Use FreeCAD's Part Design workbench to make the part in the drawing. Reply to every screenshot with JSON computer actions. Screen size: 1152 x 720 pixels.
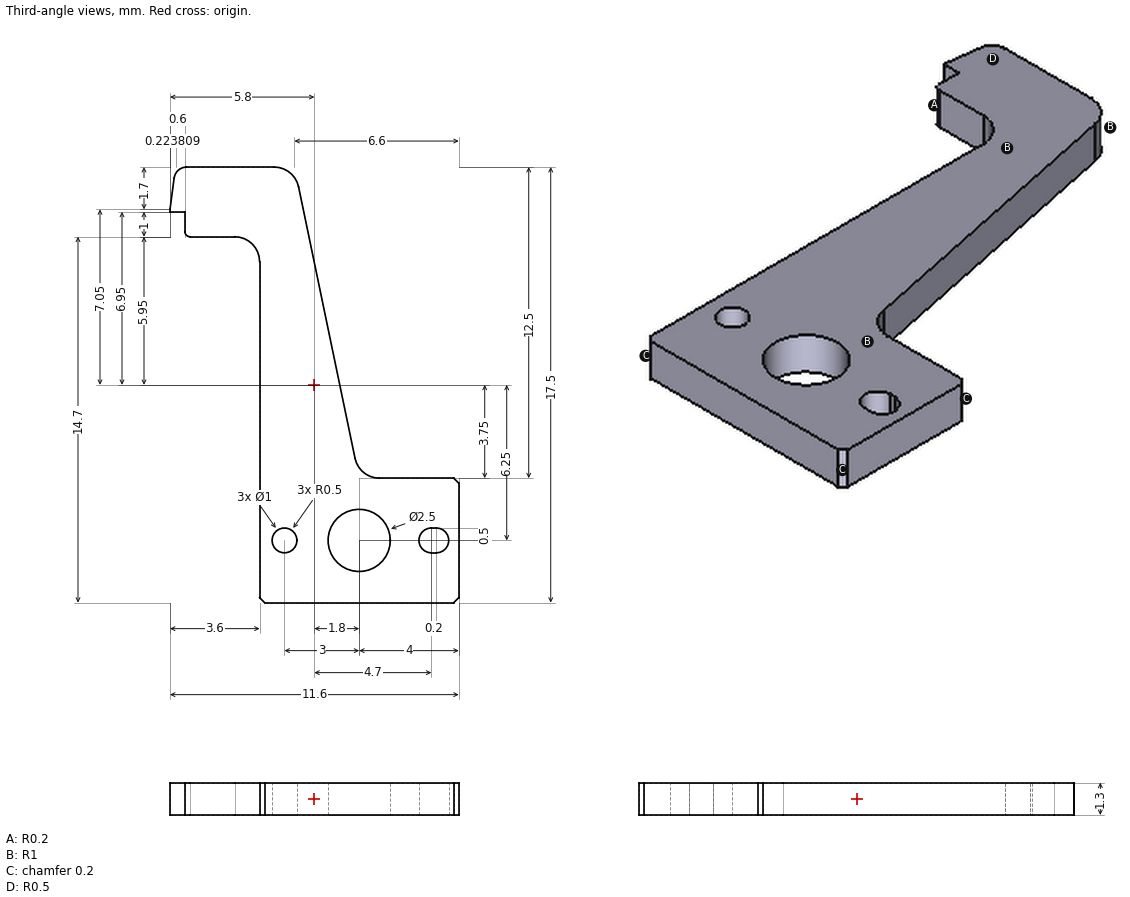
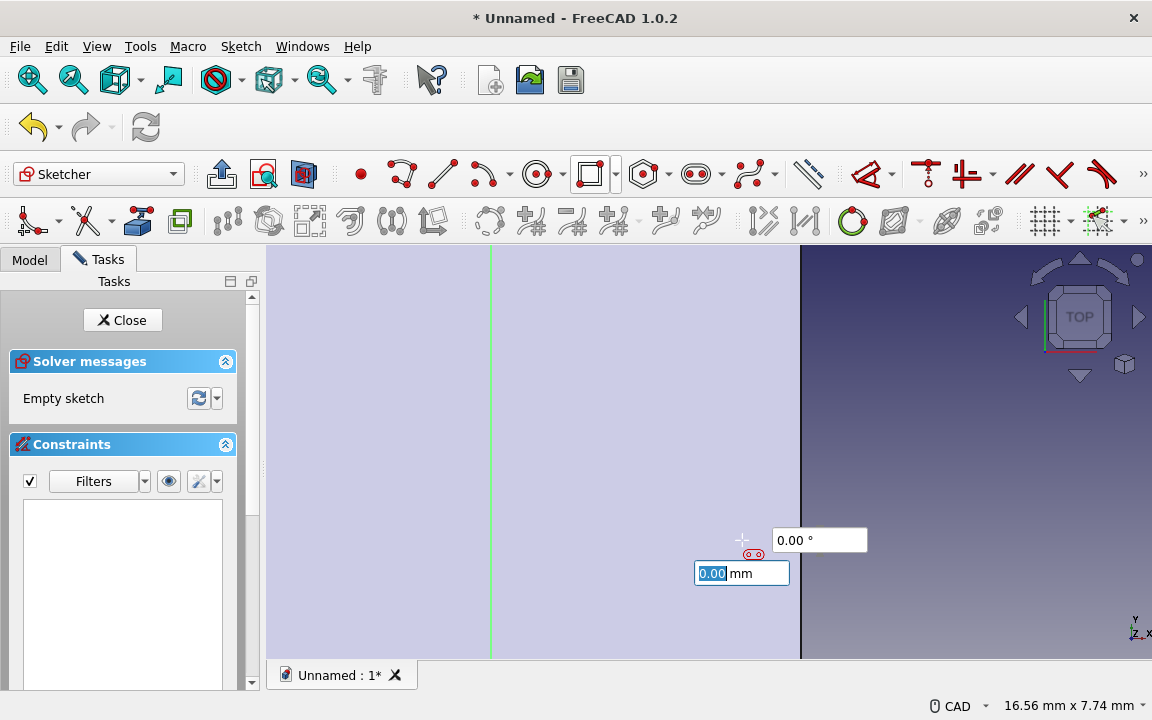
{"action": "scroll", "coordinate": [753, 540], "scroll_direction": "up", "scroll_amount": 2}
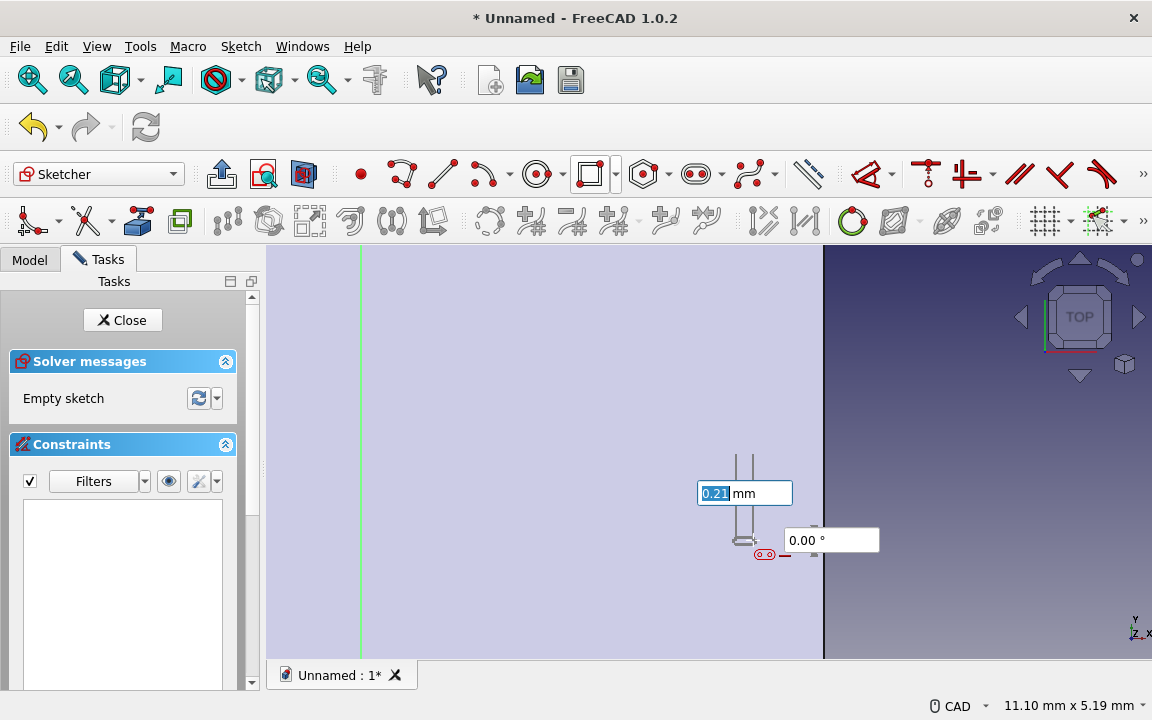
{"action": "left_click", "coordinate": [752, 540]}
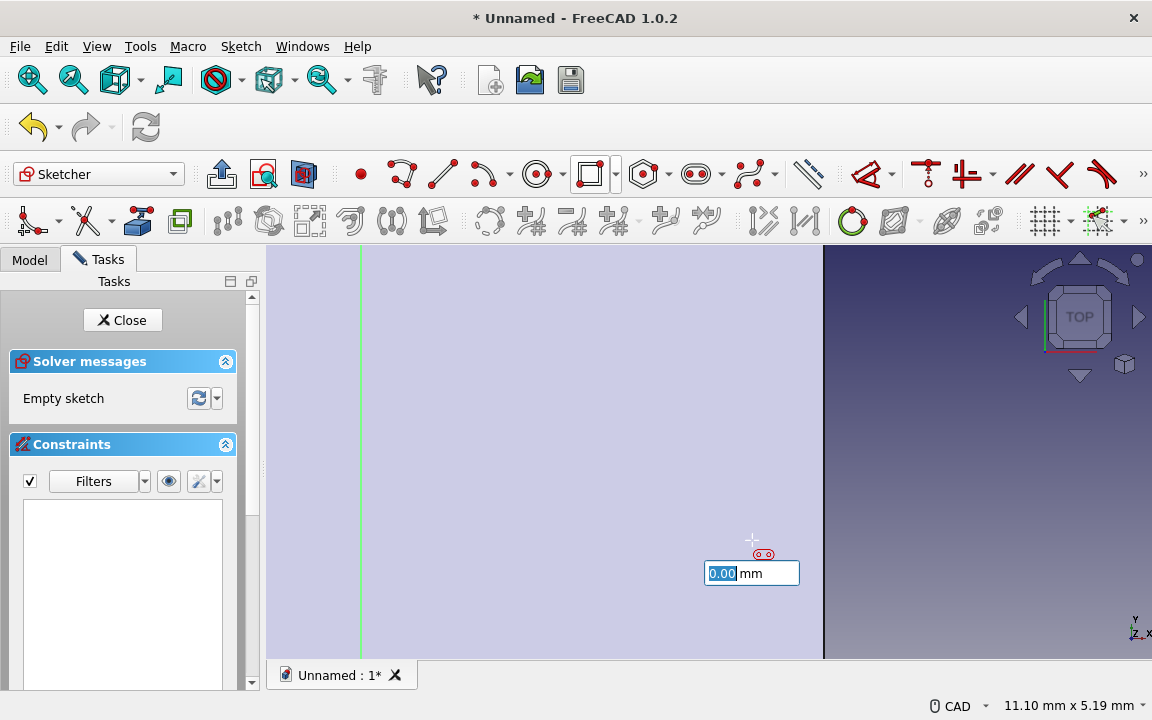
{"action": "left_click", "coordinate": [744, 500]}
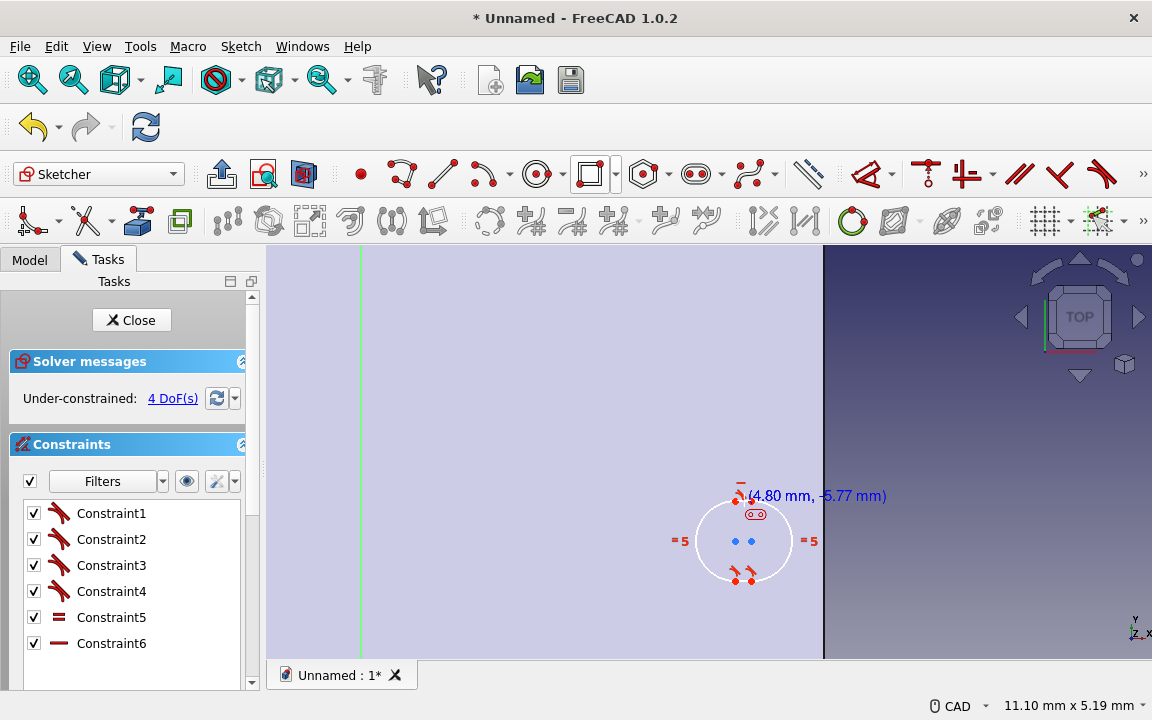
{"action": "left_click", "coordinate": [536, 174]}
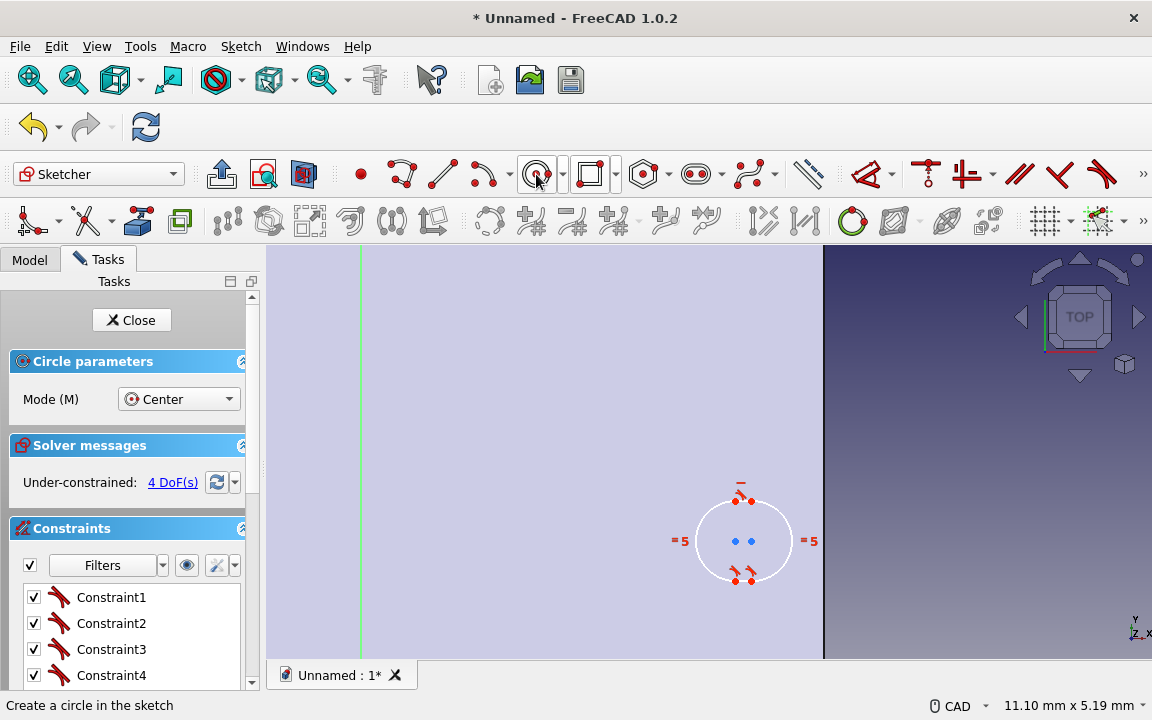
{"action": "left_click", "coordinate": [505, 540]}
{"action": "left_click", "coordinate": [575, 469]}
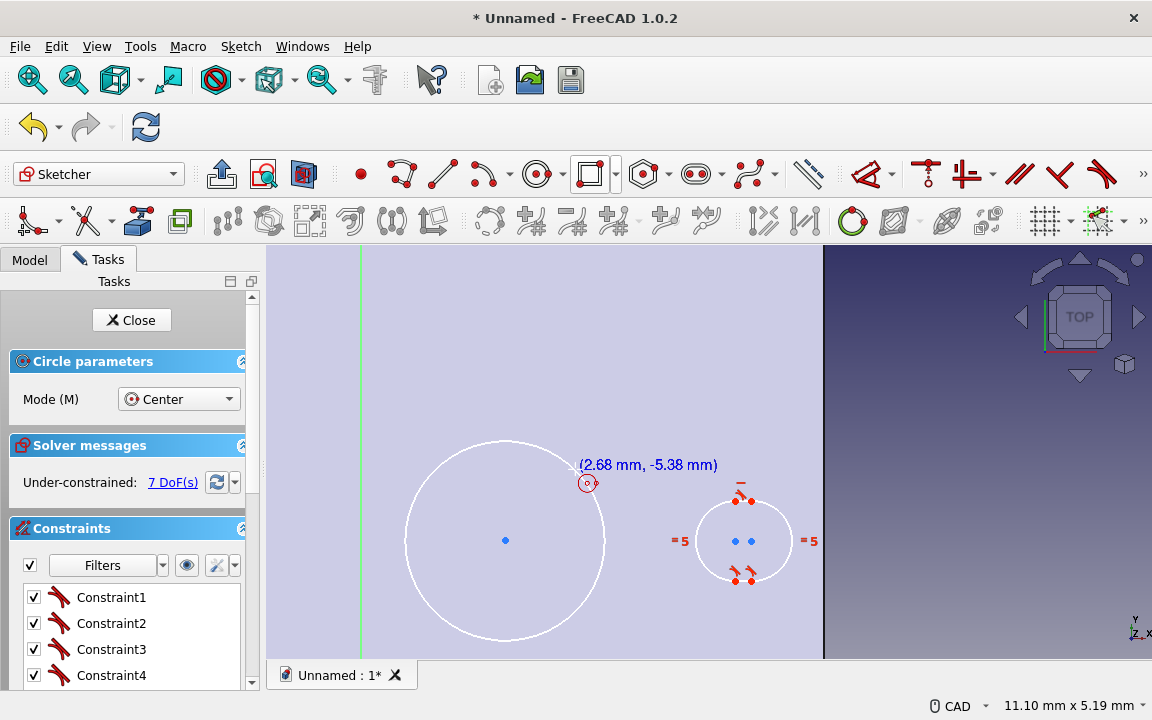
{"action": "scroll", "coordinate": [748, 543], "scroll_direction": "down", "scroll_amount": 4}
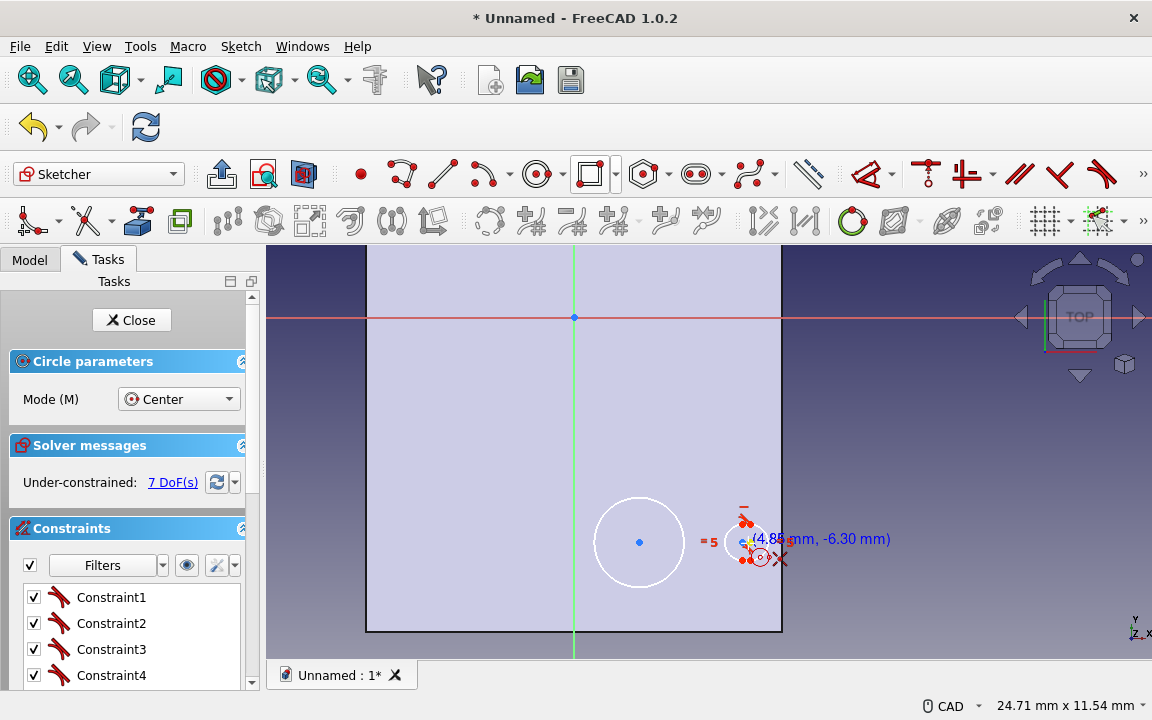
{"action": "scroll", "coordinate": [531, 542], "scroll_direction": "up", "scroll_amount": 2}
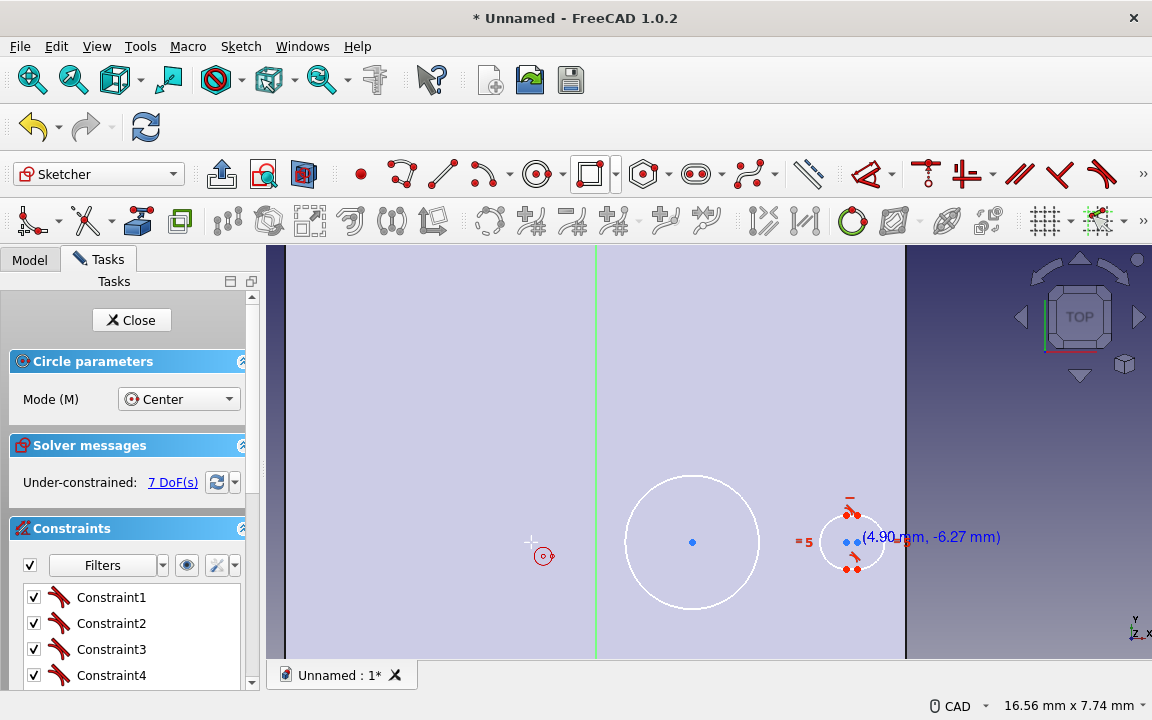
{"action": "left_click", "coordinate": [532, 541]}
{"action": "left_click", "coordinate": [550, 523]}
{"action": "key", "text": "Escape"}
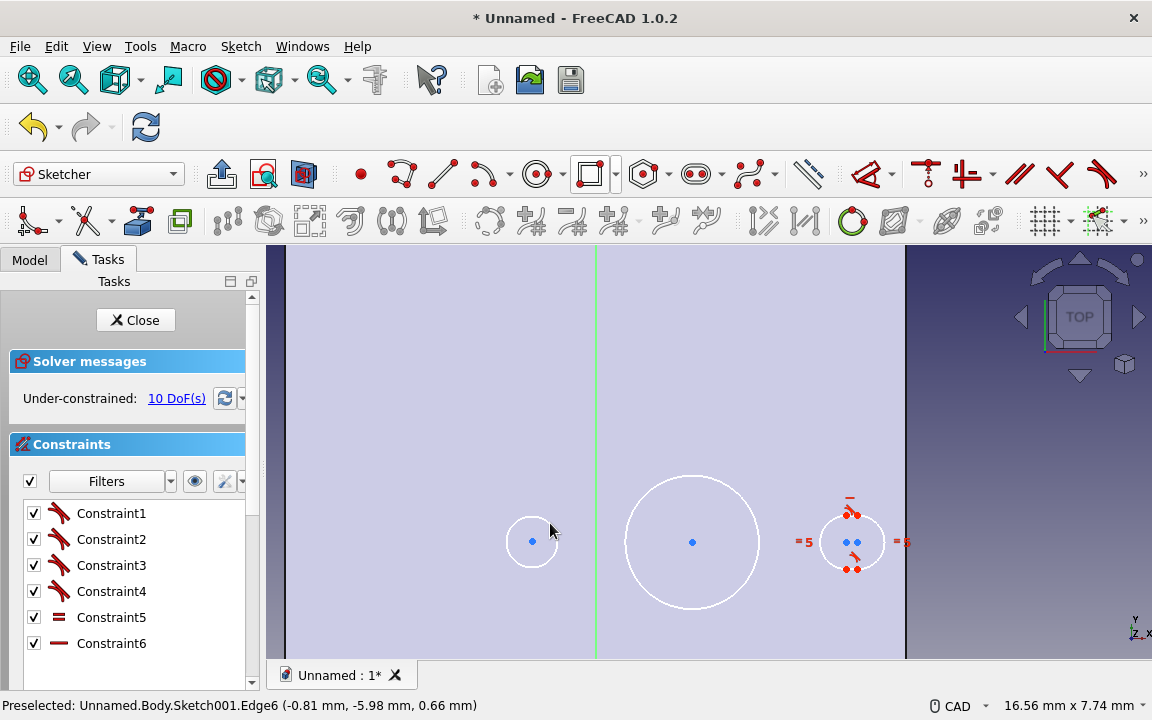
{"action": "left_click", "coordinate": [692, 542]}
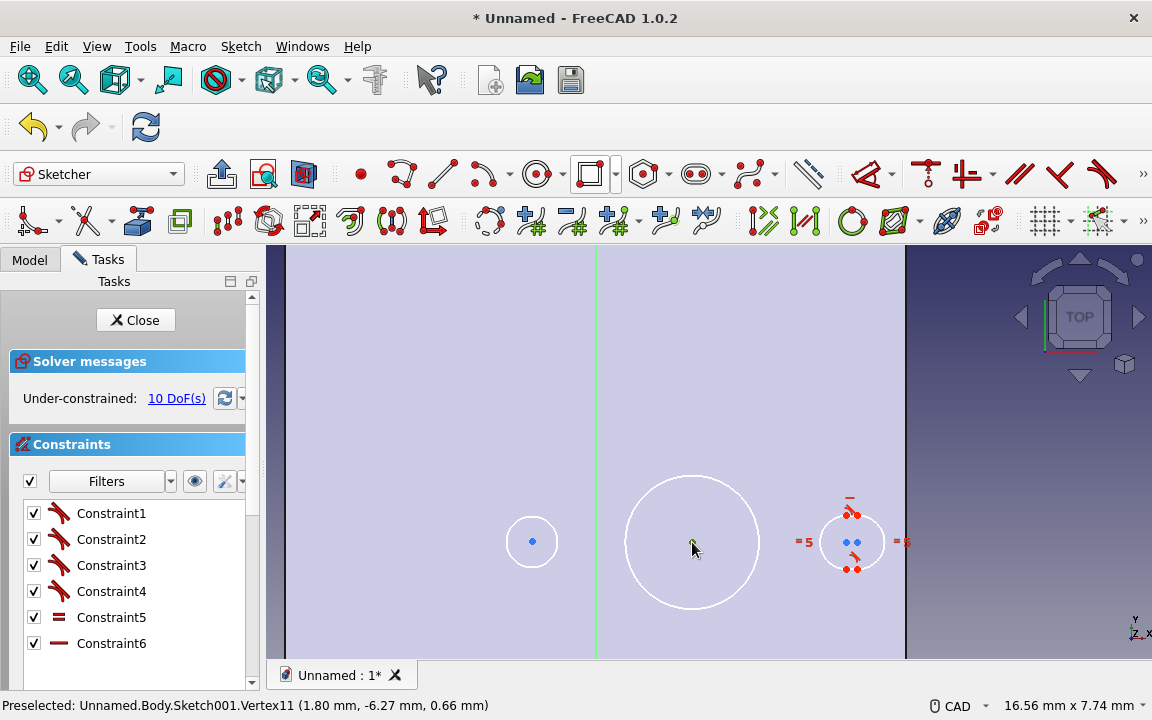
{"action": "left_click", "coordinate": [532, 542]}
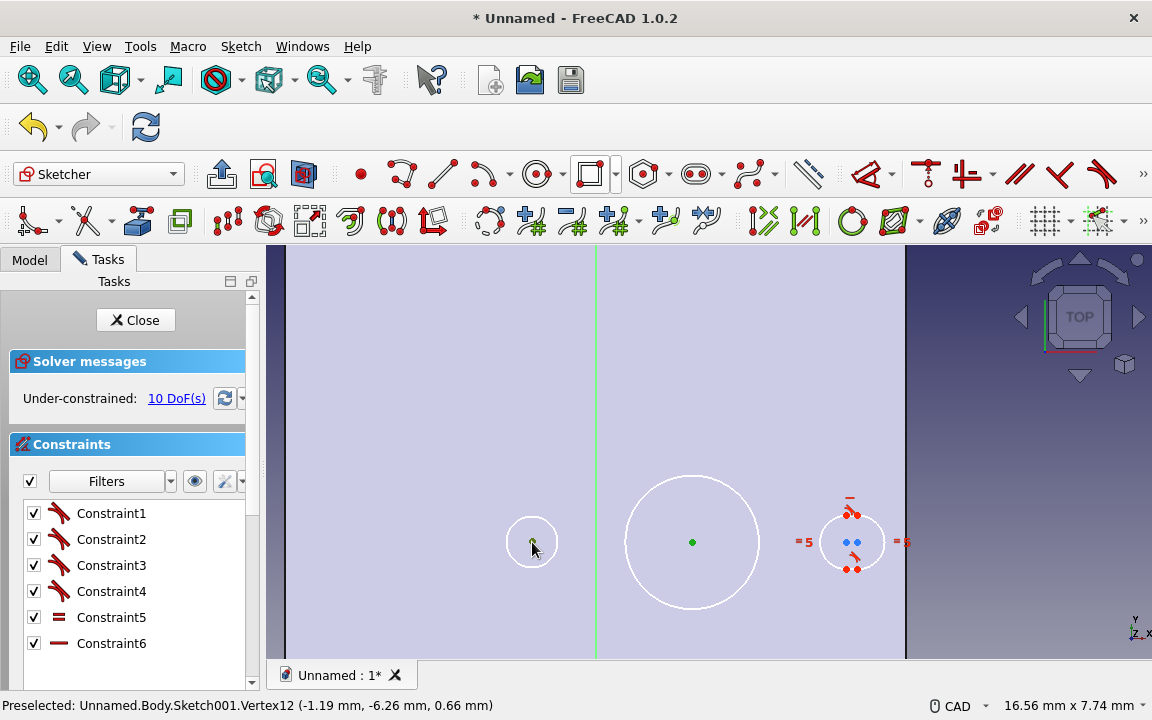
{"action": "key", "text": "h"}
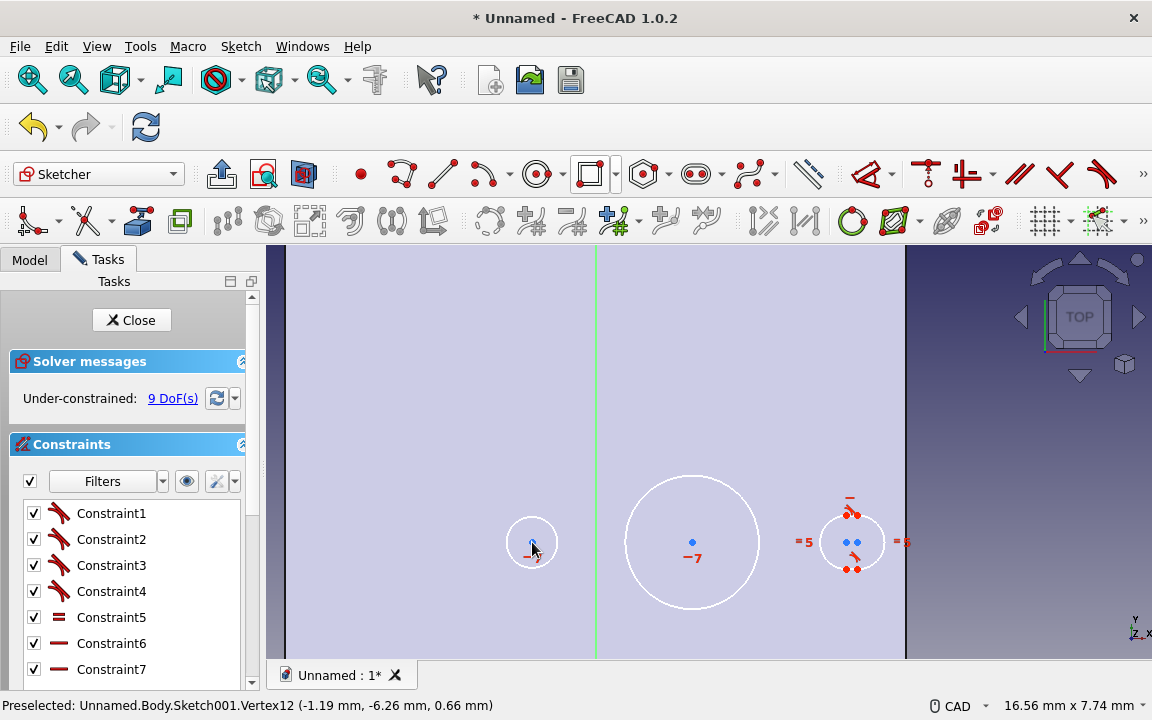
{"action": "key", "text": "d"}